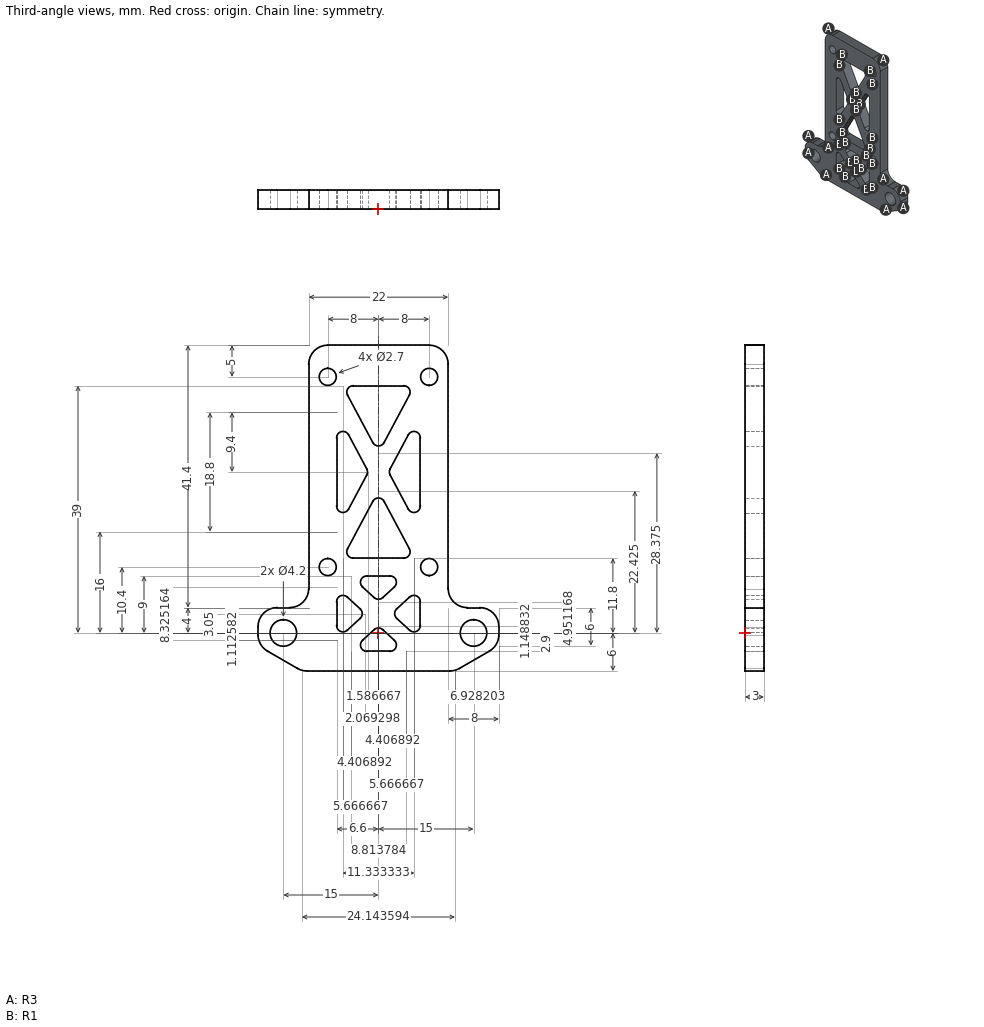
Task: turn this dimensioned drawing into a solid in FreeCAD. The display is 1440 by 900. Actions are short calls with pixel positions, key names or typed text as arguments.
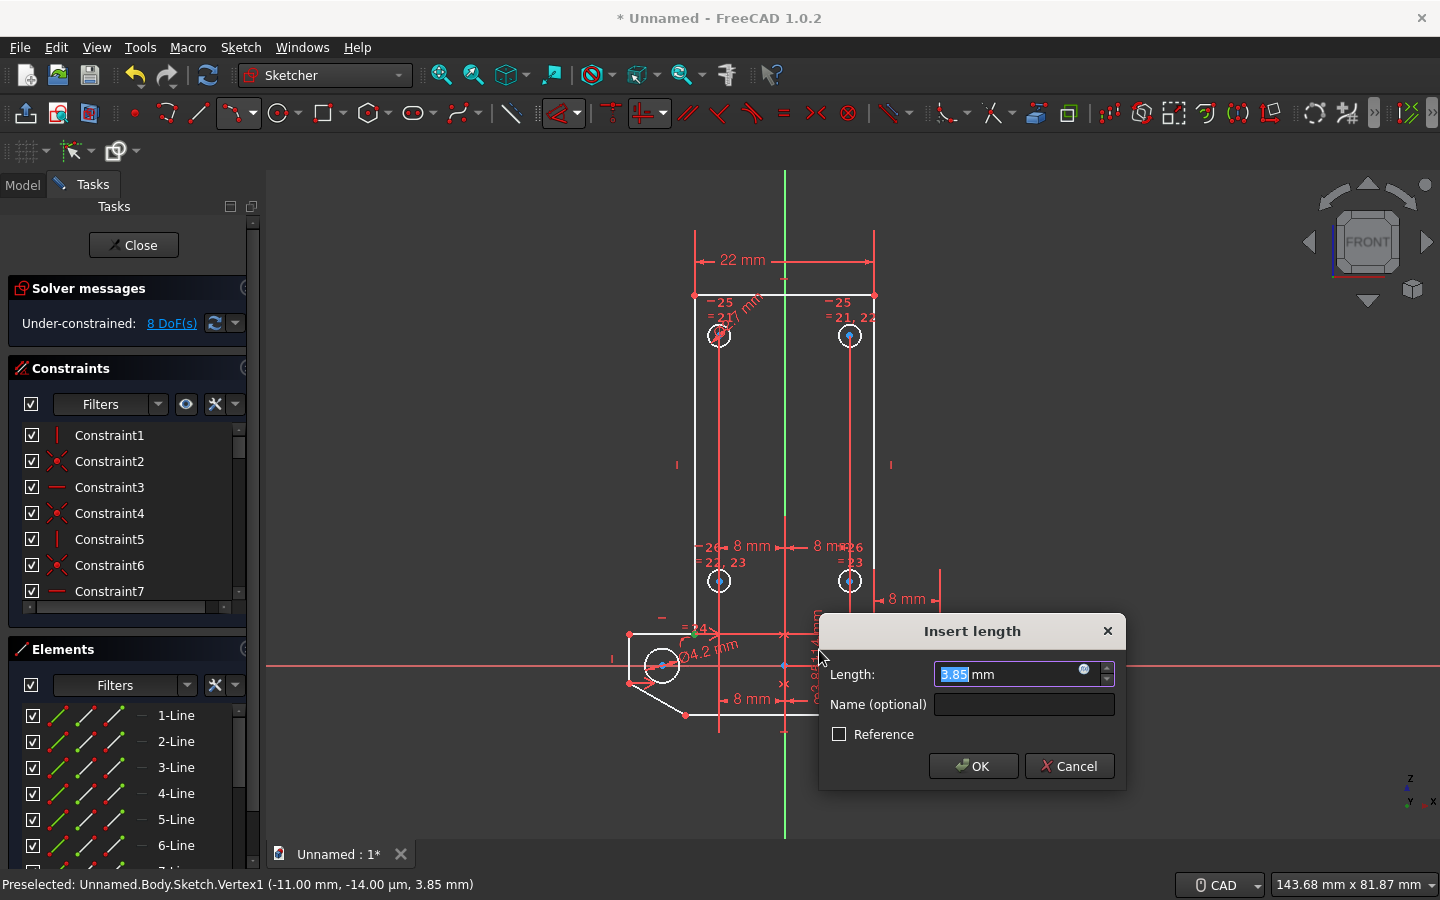
text(4)
key(Return)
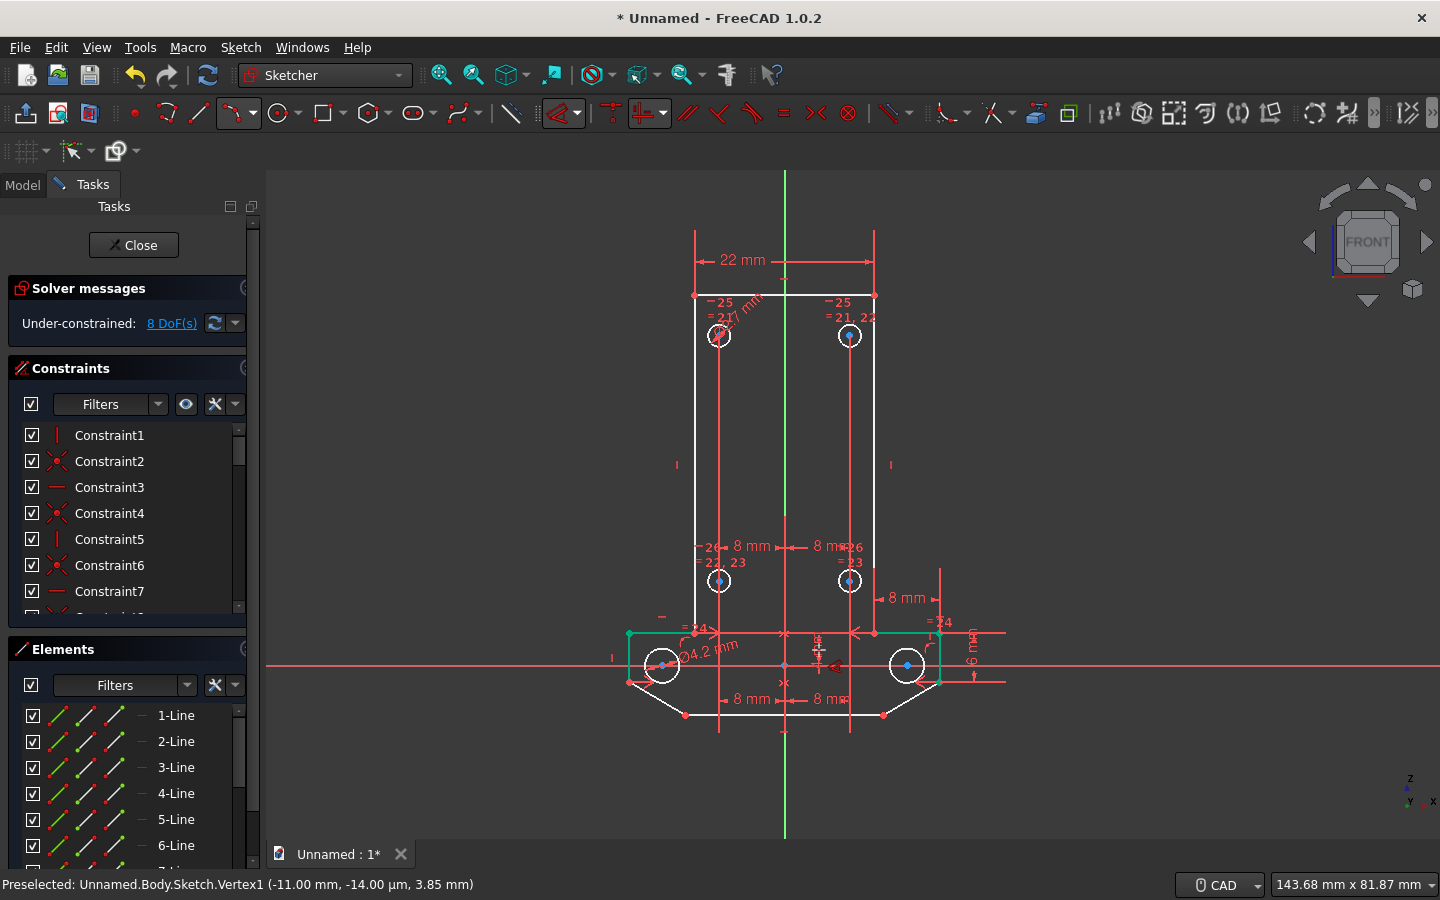
click(884, 715)
click(751, 679)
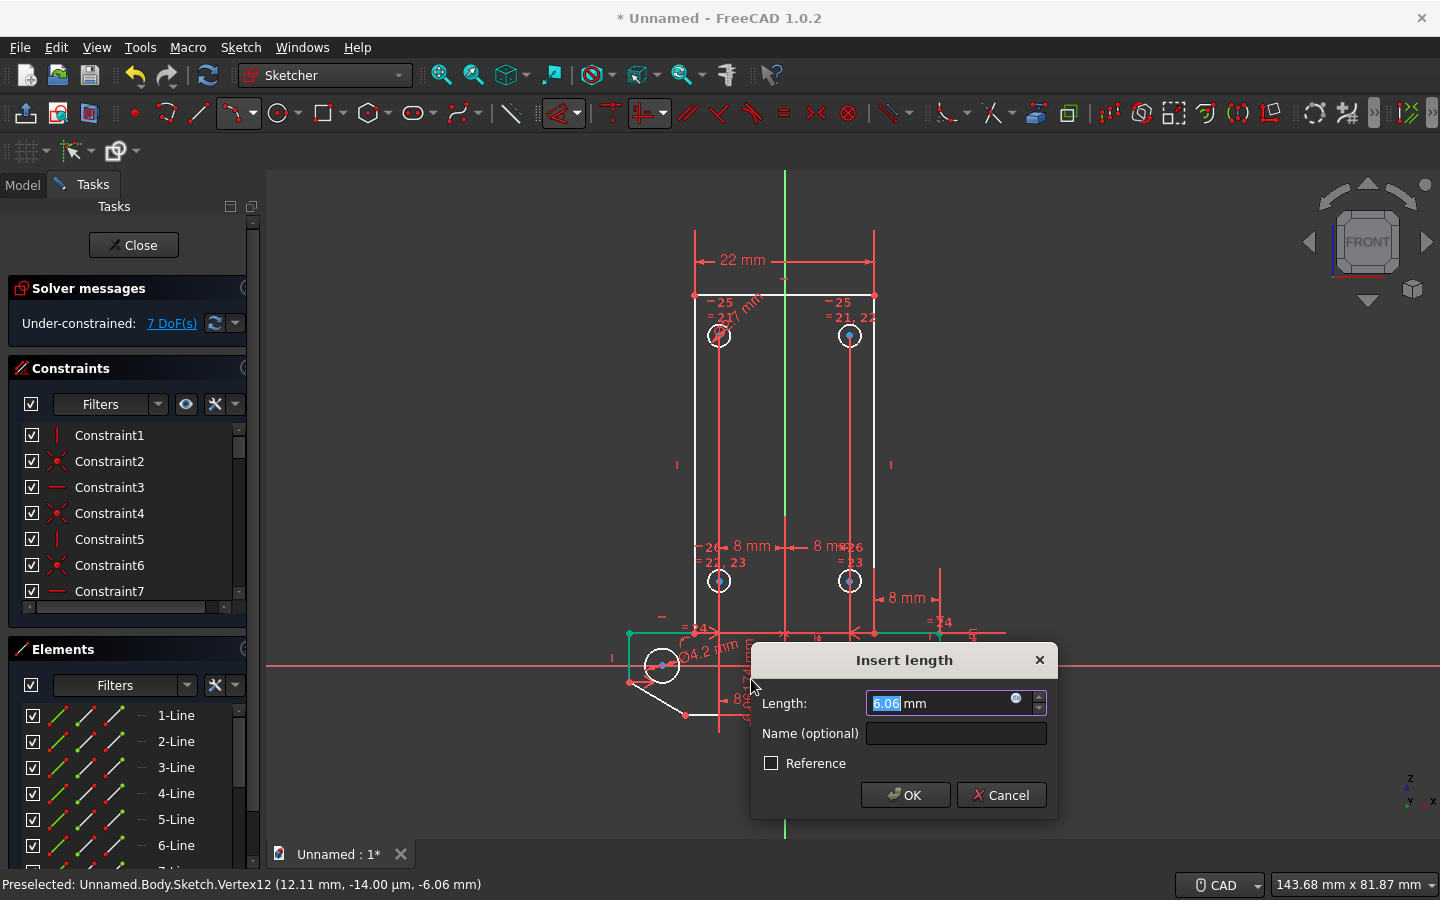
text(6)
key(Return)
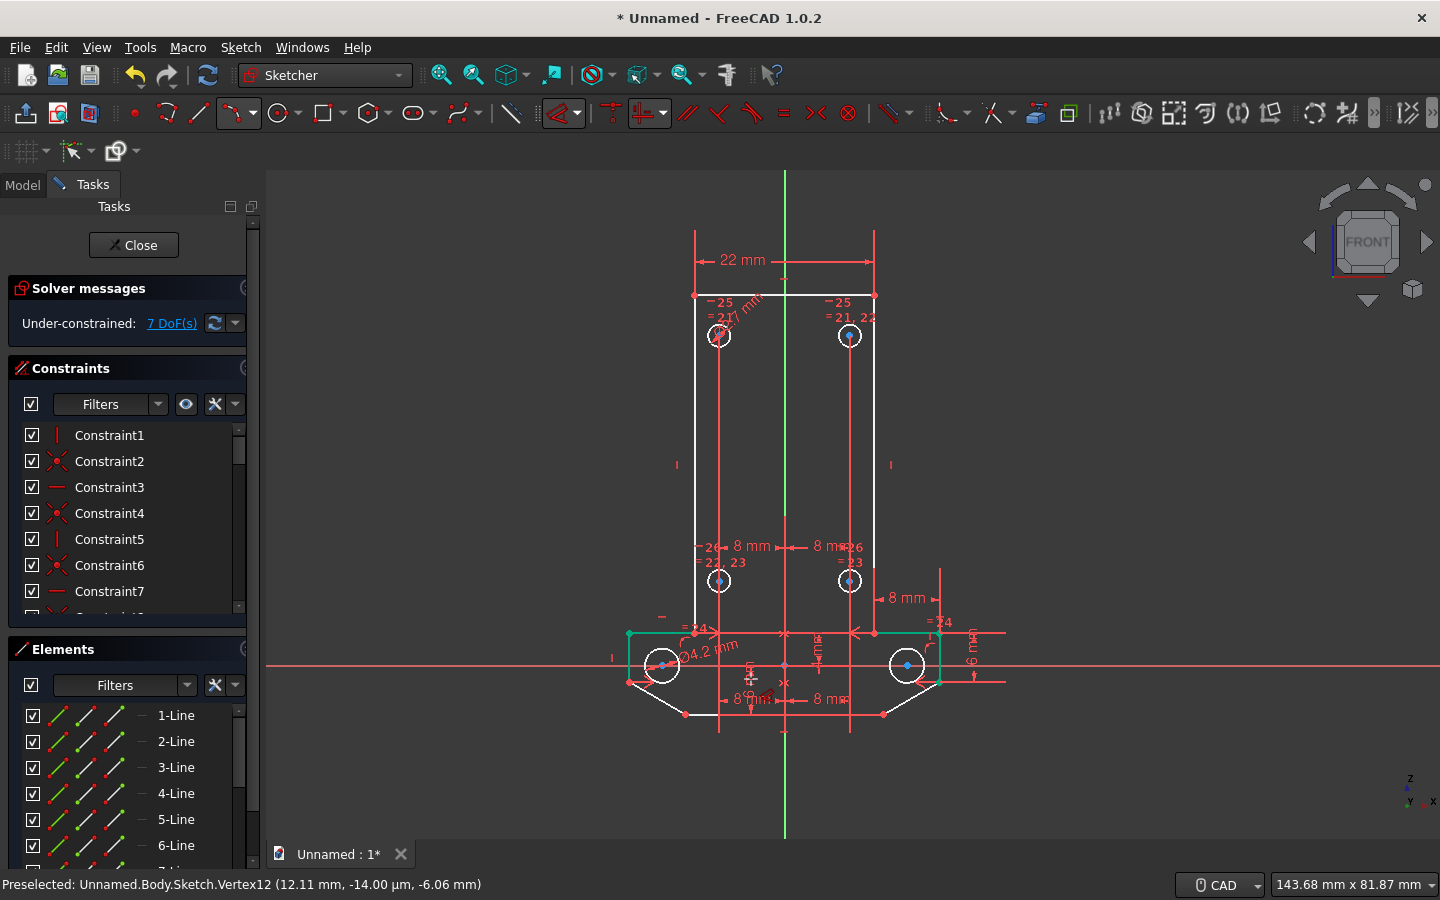
click(662, 666)
click(723, 632)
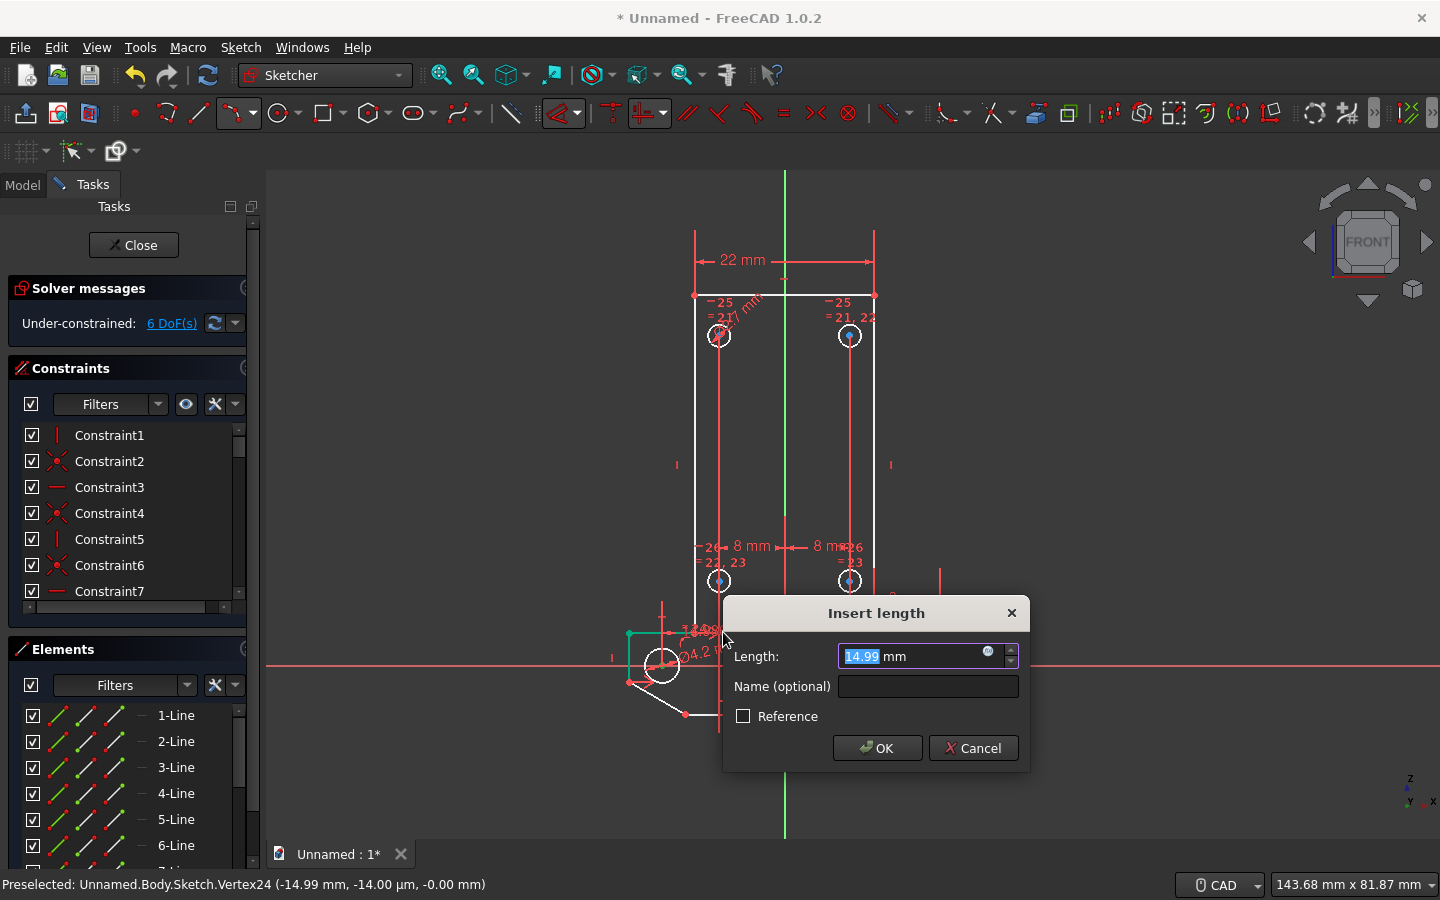
text(15)
key(Return)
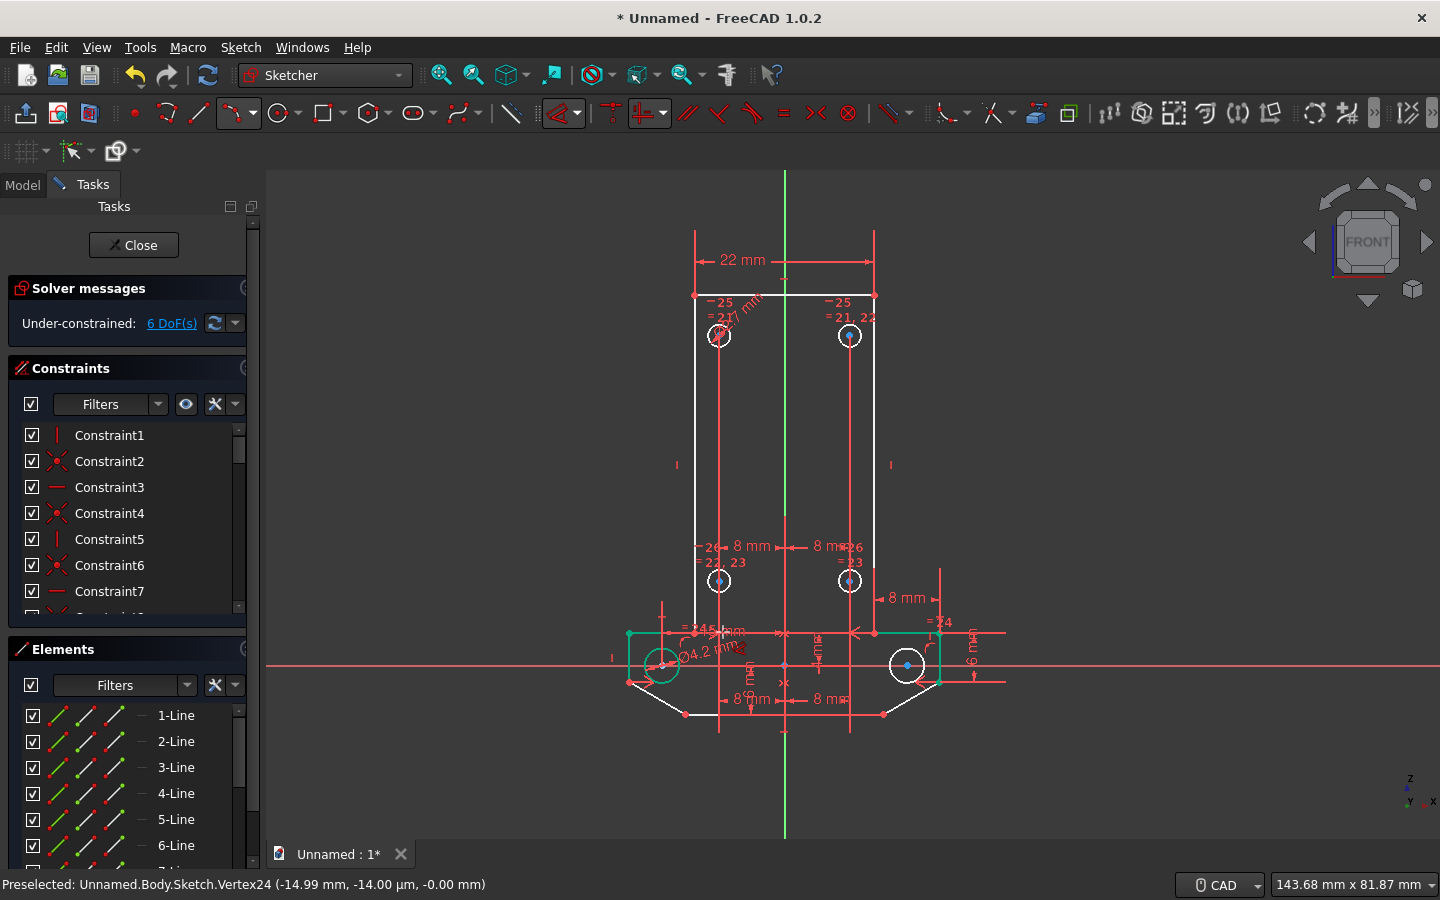
click(907, 666)
click(818, 608)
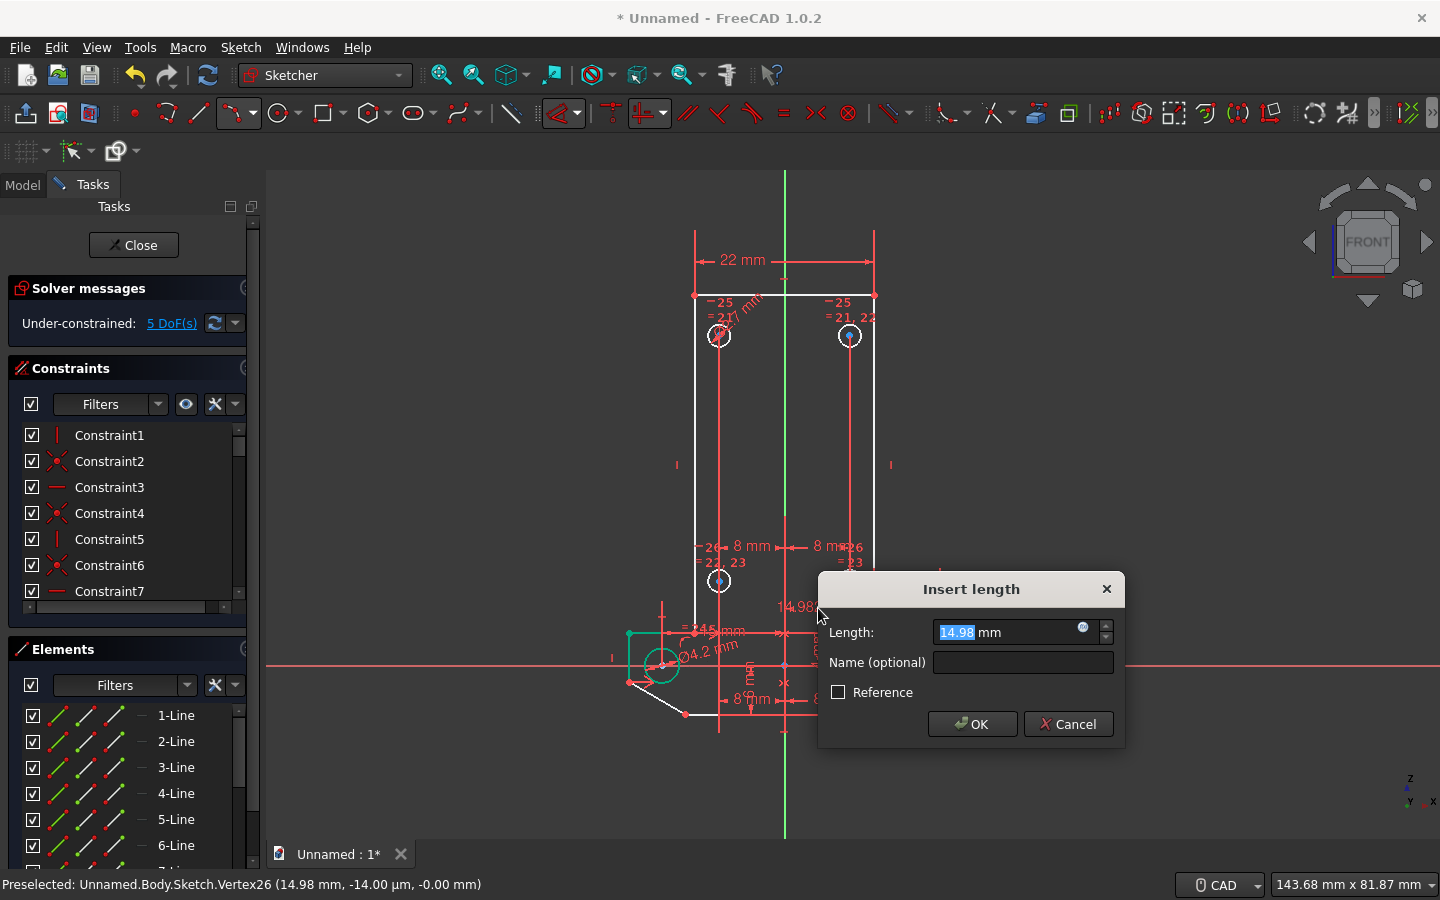
text(15)
key(Return)